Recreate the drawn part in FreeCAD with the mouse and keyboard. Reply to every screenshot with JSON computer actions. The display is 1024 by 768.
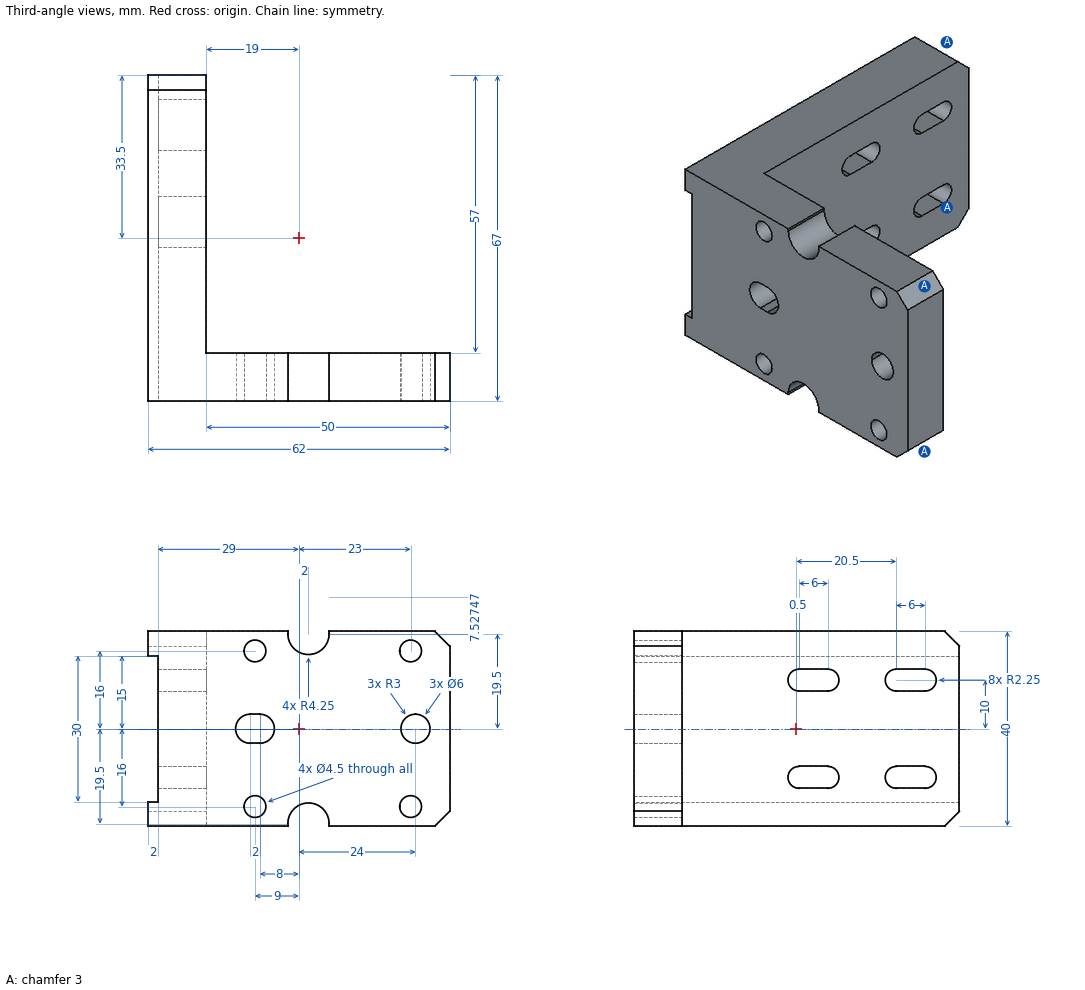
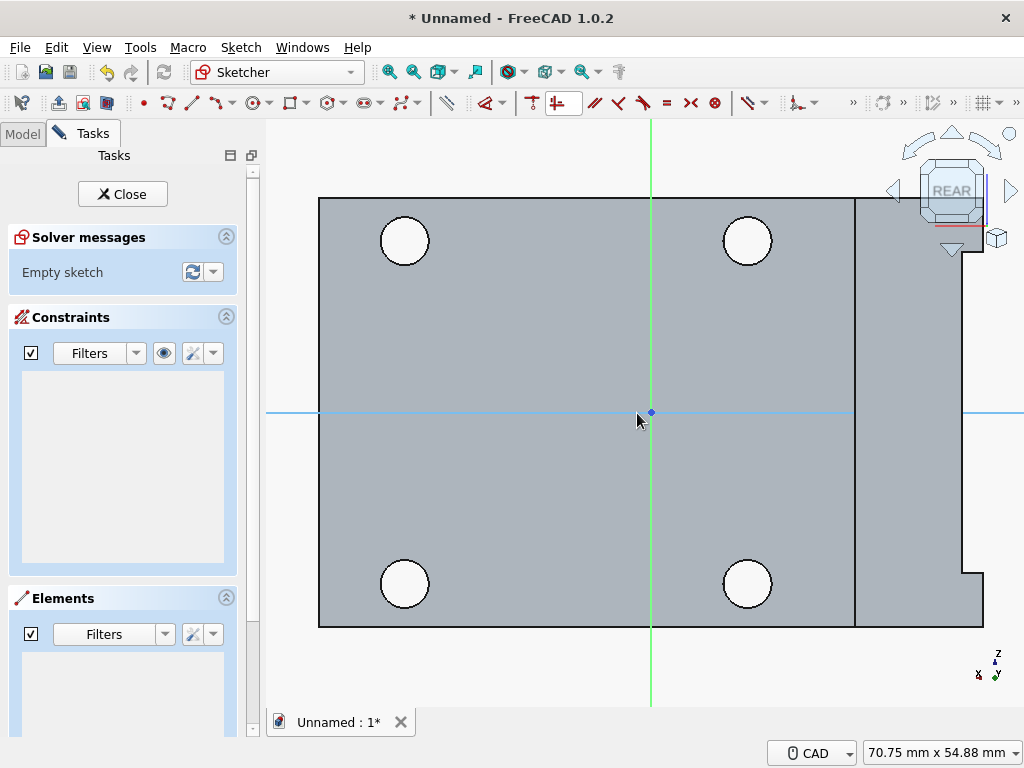
{"action": "left_click", "coordinate": [364, 104]}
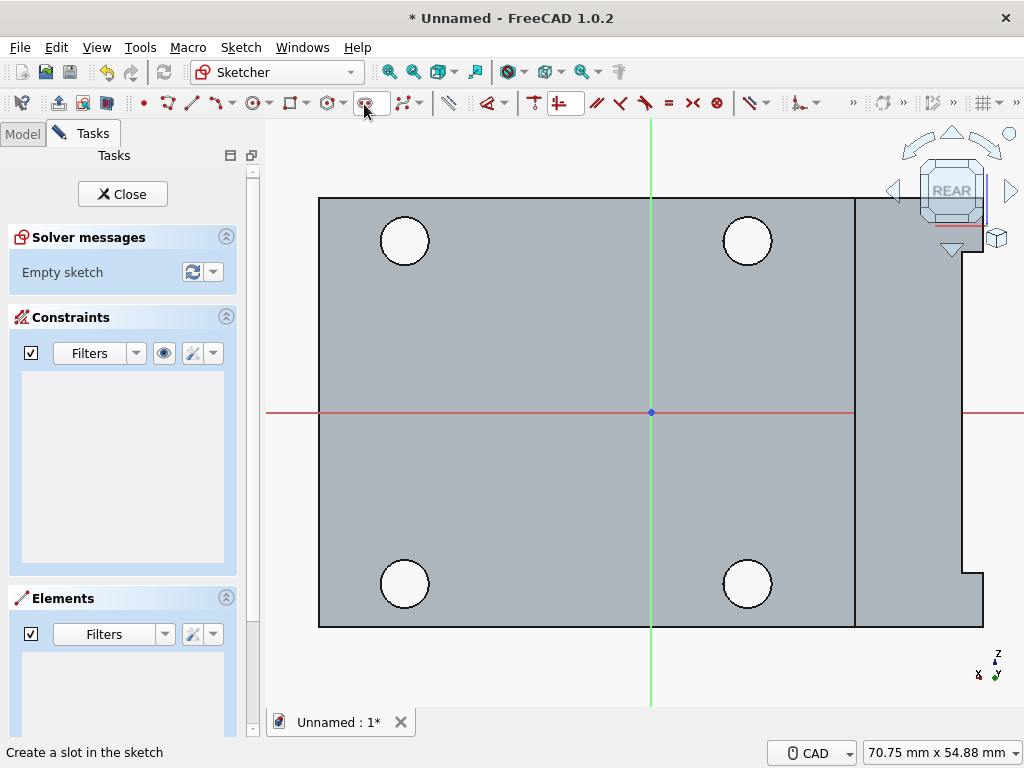
{"action": "left_click", "coordinate": [737, 413]}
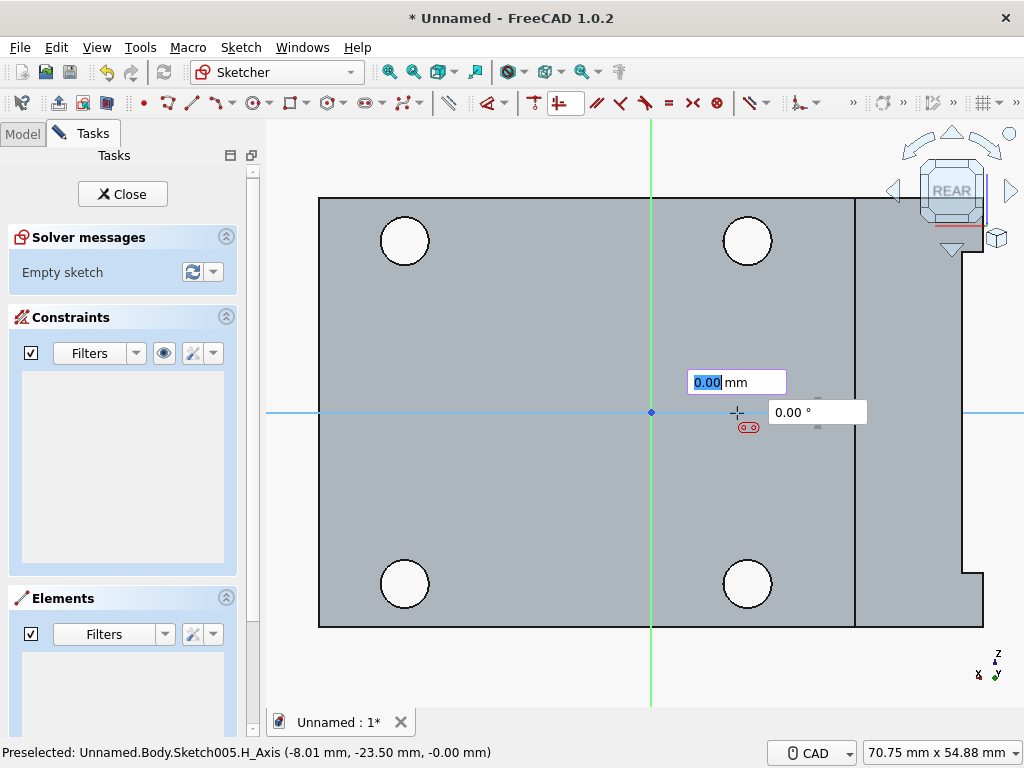
{"action": "left_click", "coordinate": [758, 404]}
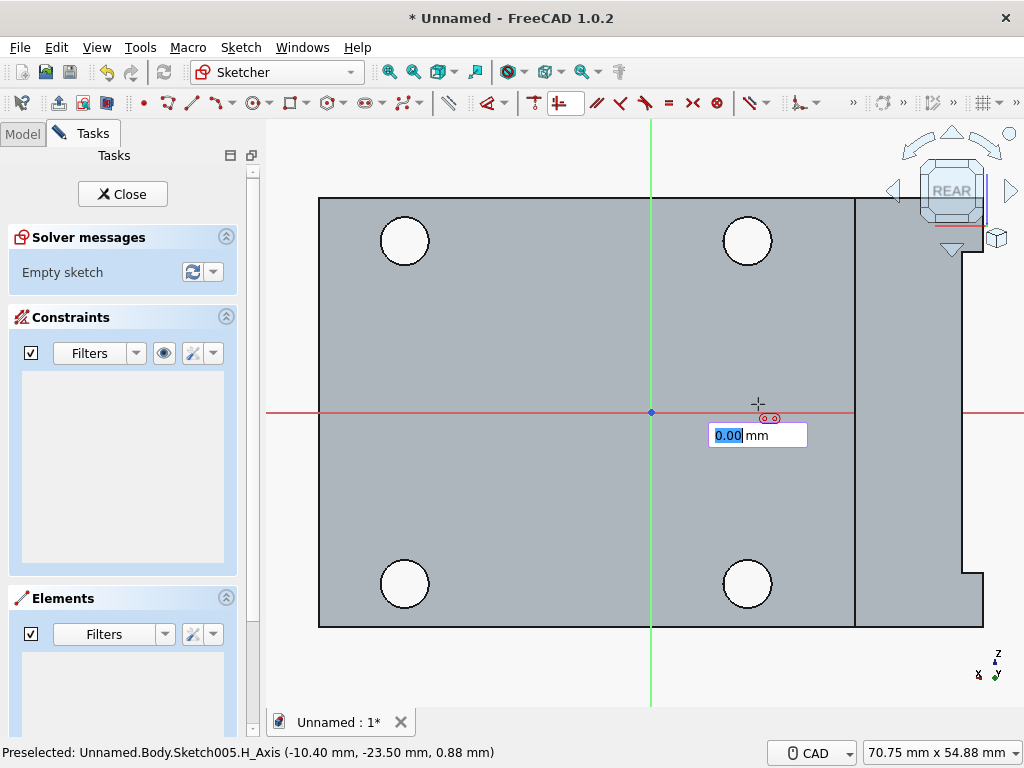
{"action": "left_click", "coordinate": [748, 445]}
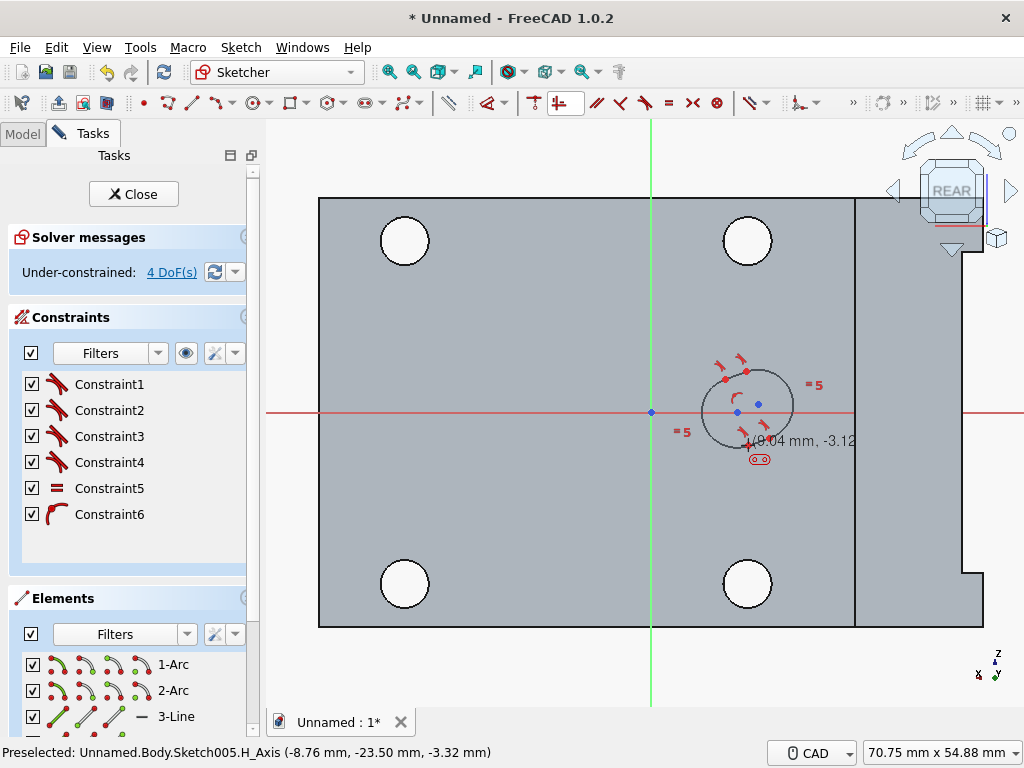
{"action": "left_click", "coordinate": [254, 104]}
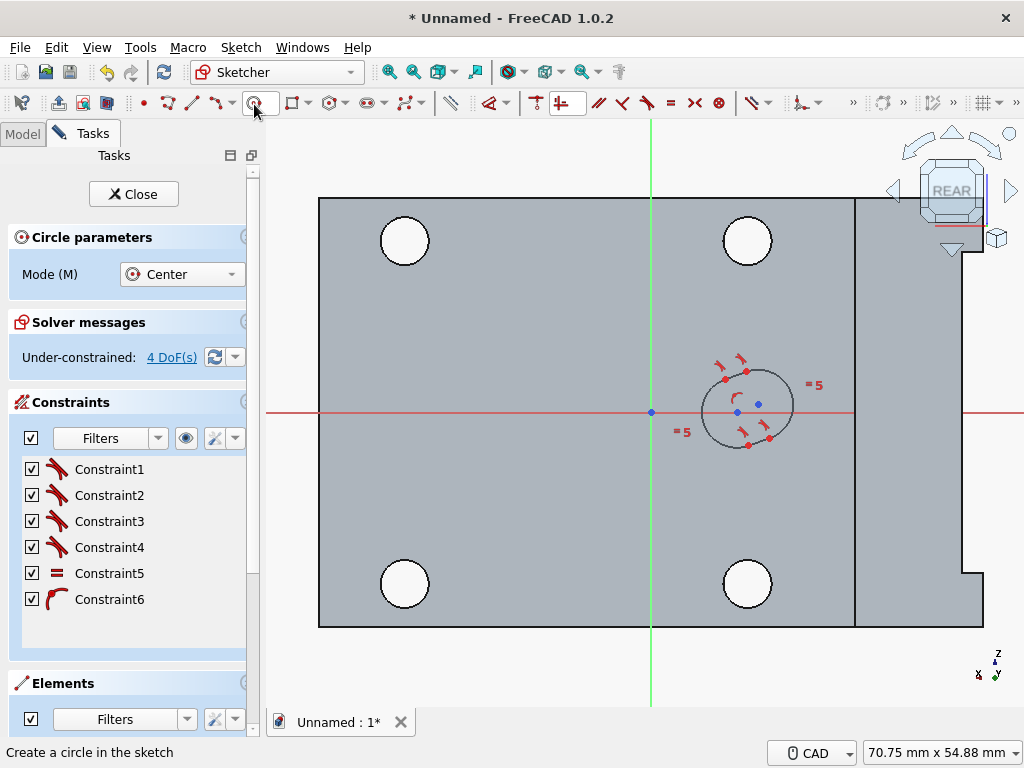
{"action": "left_click", "coordinate": [394, 413]}
{"action": "mouse_move", "coordinate": [417, 390]}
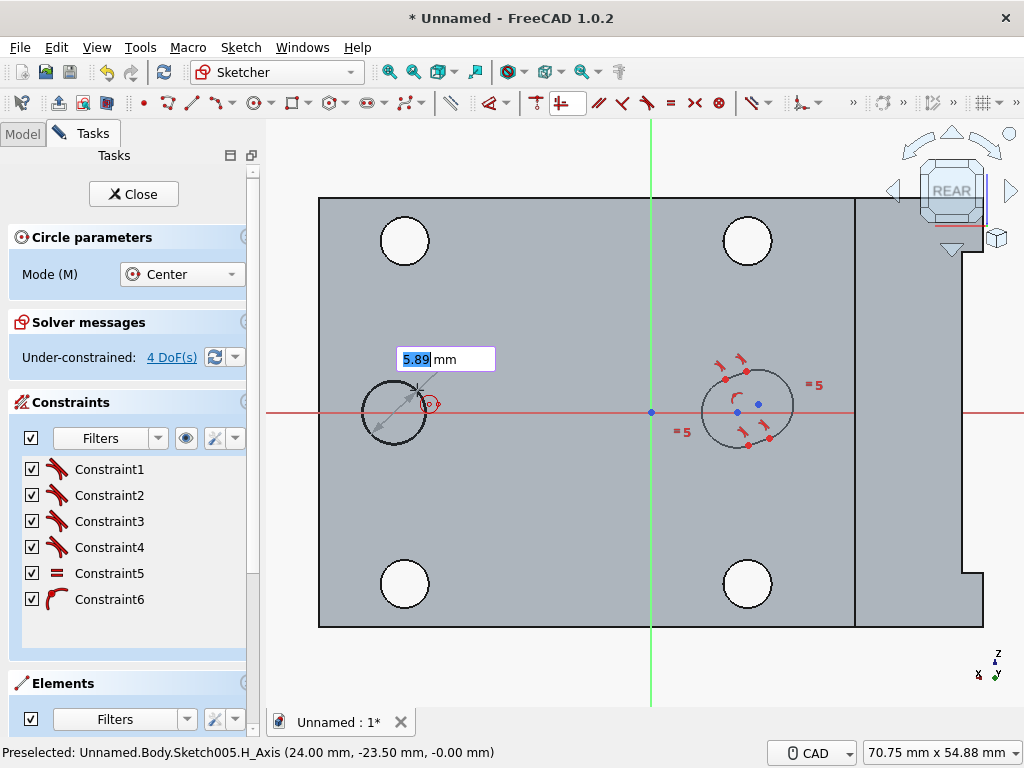
{"action": "type", "text": "6"}
{"action": "key", "text": "Return"}
{"action": "key", "text": "Escape"}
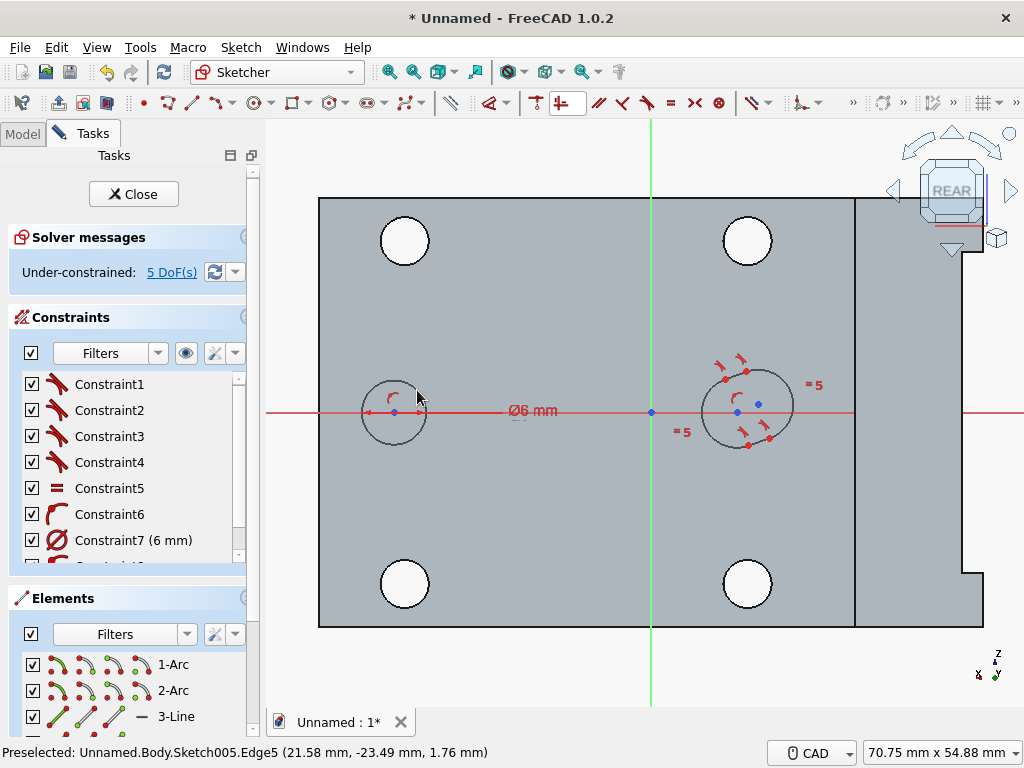
{"action": "scroll", "coordinate": [736, 376], "scroll_direction": "up", "scroll_amount": 2}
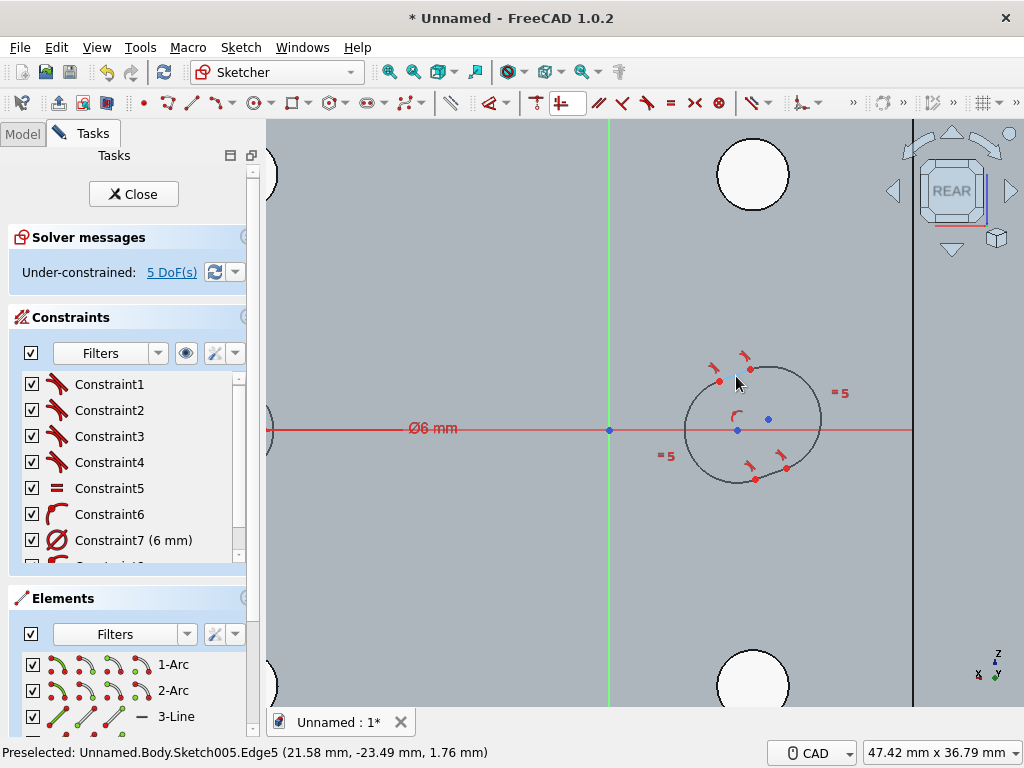
{"action": "left_click", "coordinate": [735, 375]}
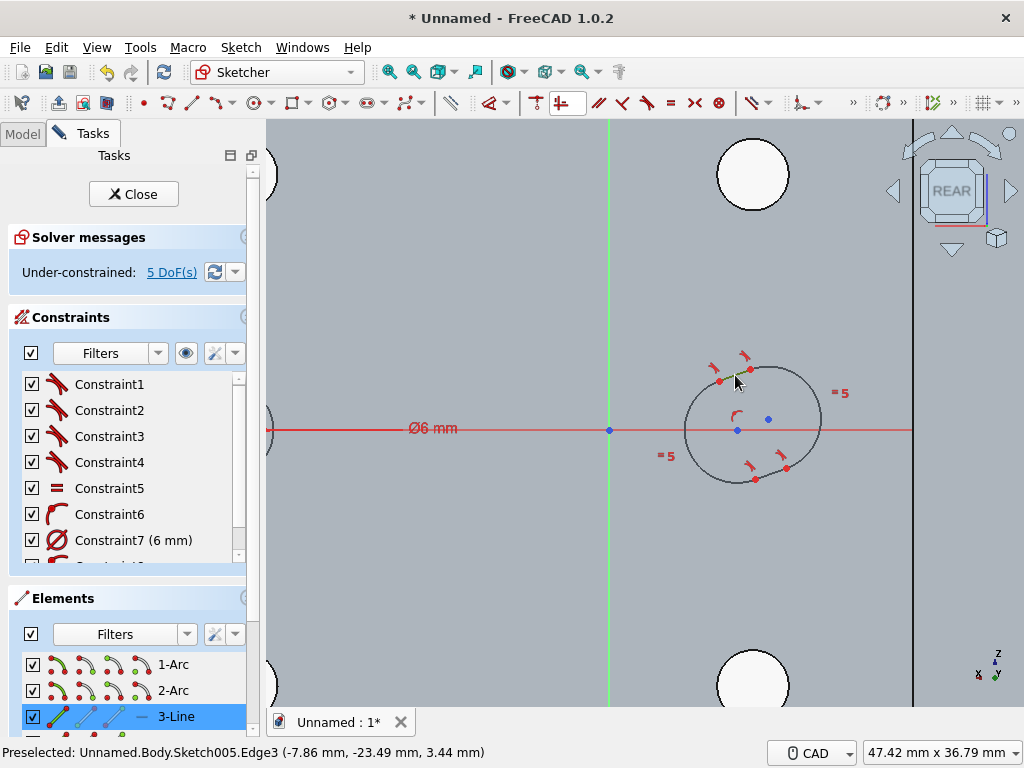
{"action": "key", "text": "h"}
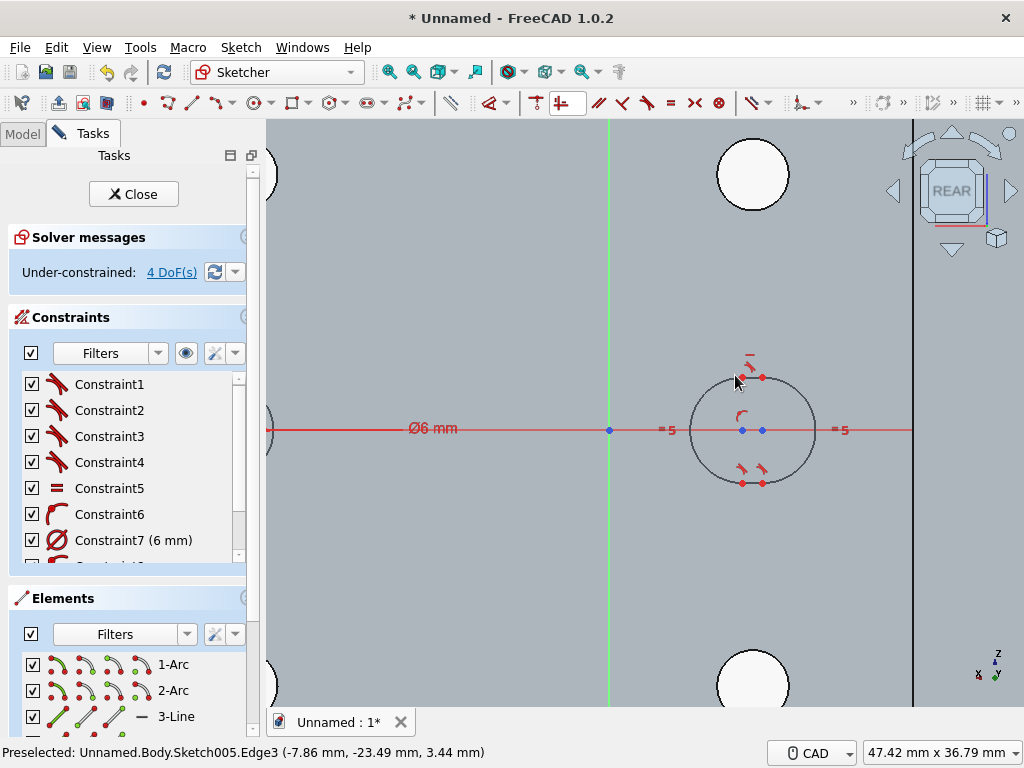
{"action": "left_click", "coordinate": [490, 104]}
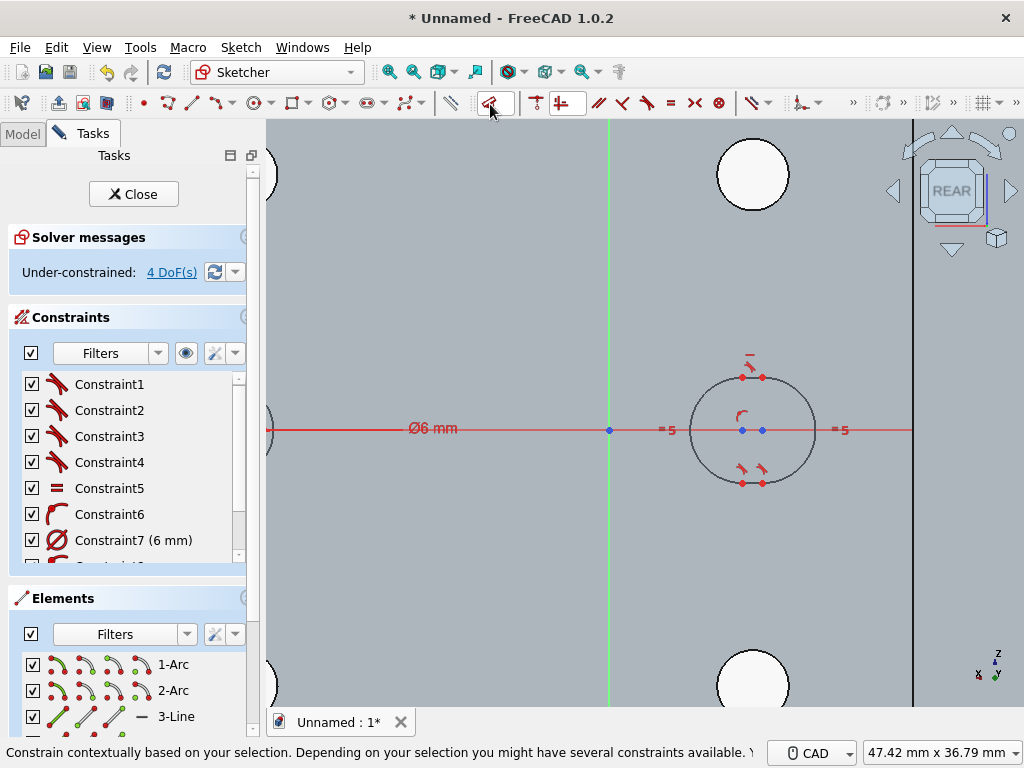
{"action": "left_click", "coordinate": [700, 399]}
{"action": "left_click", "coordinate": [674, 380]}